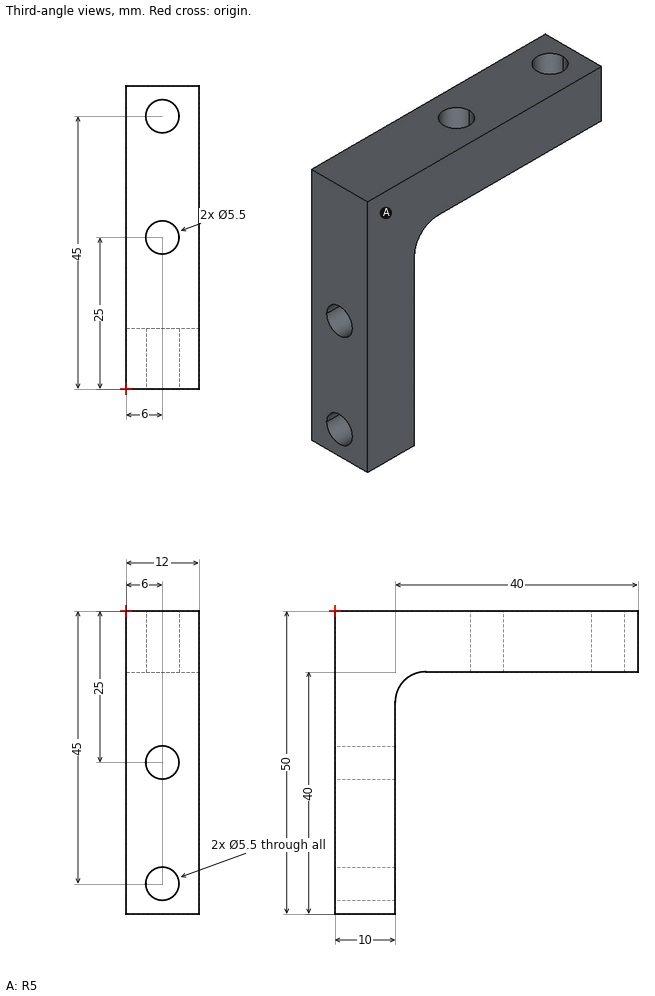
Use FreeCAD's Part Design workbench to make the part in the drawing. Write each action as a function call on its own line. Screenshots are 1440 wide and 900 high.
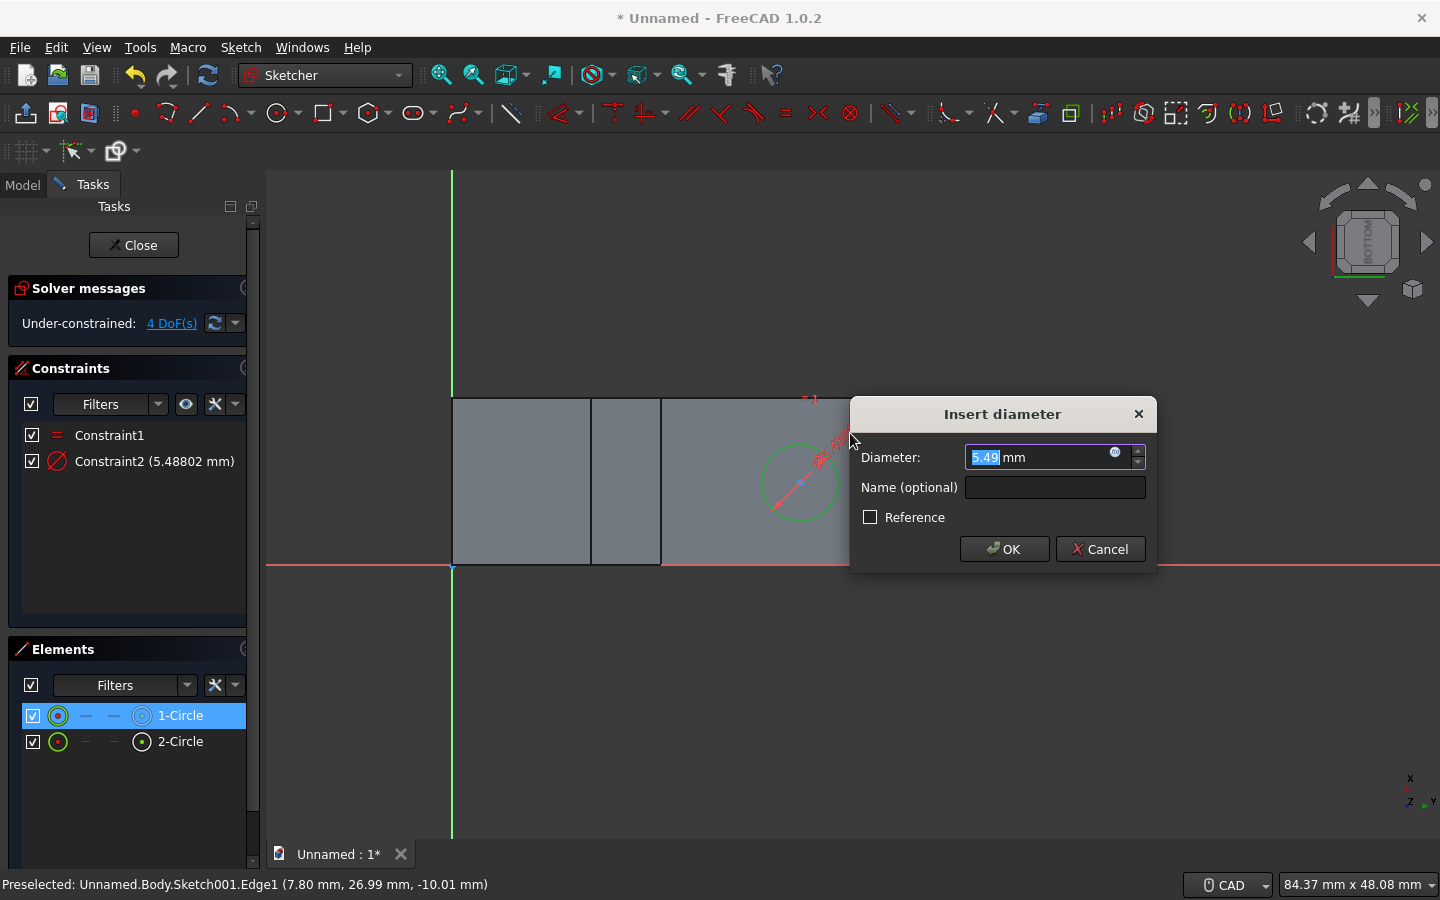
text(5.5)
key(Return)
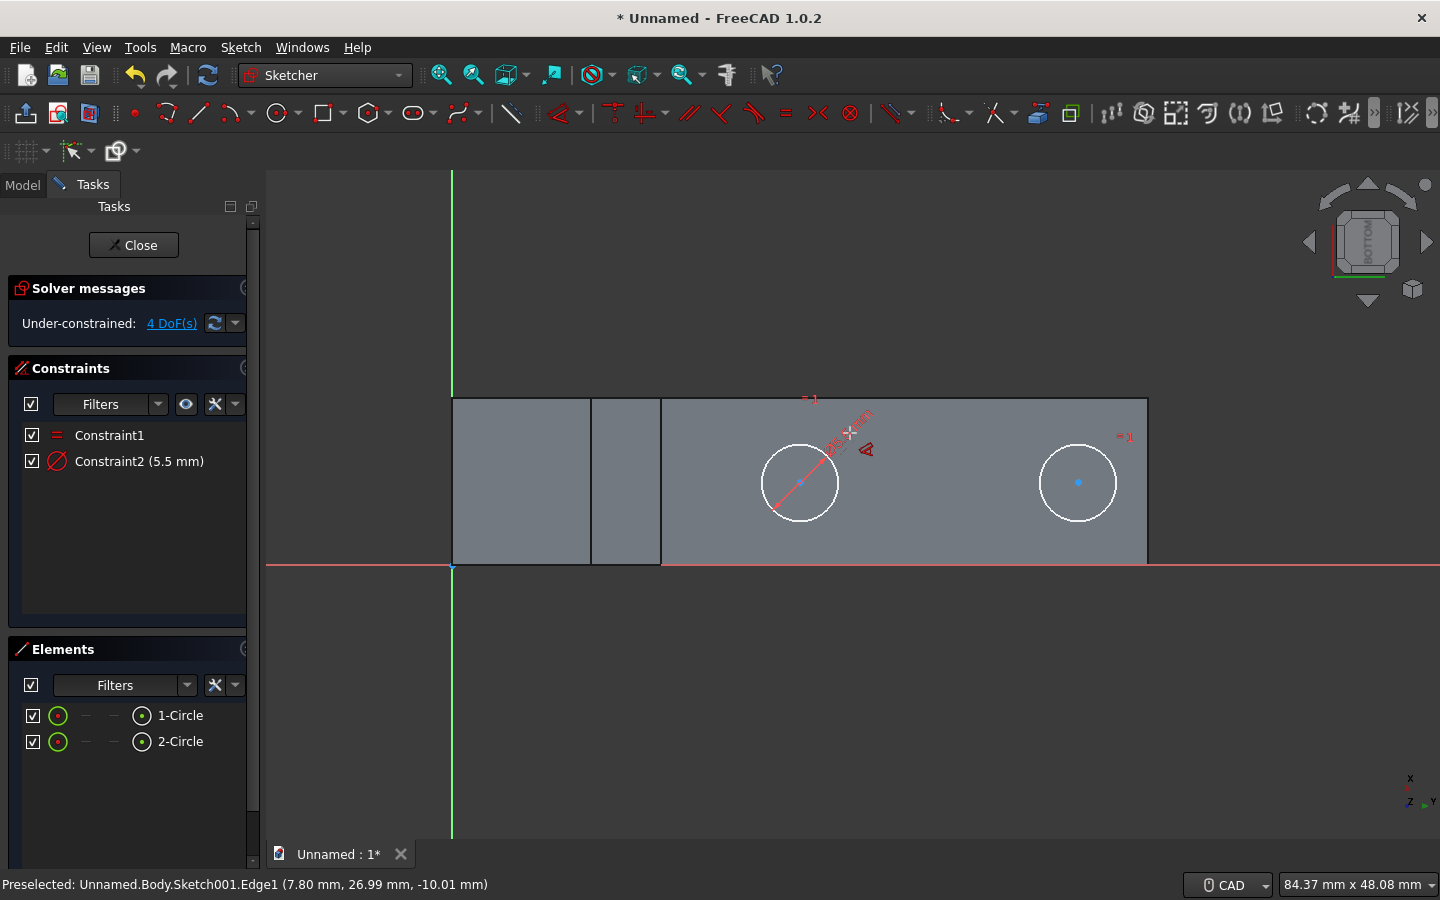
click(800, 483)
click(418, 524)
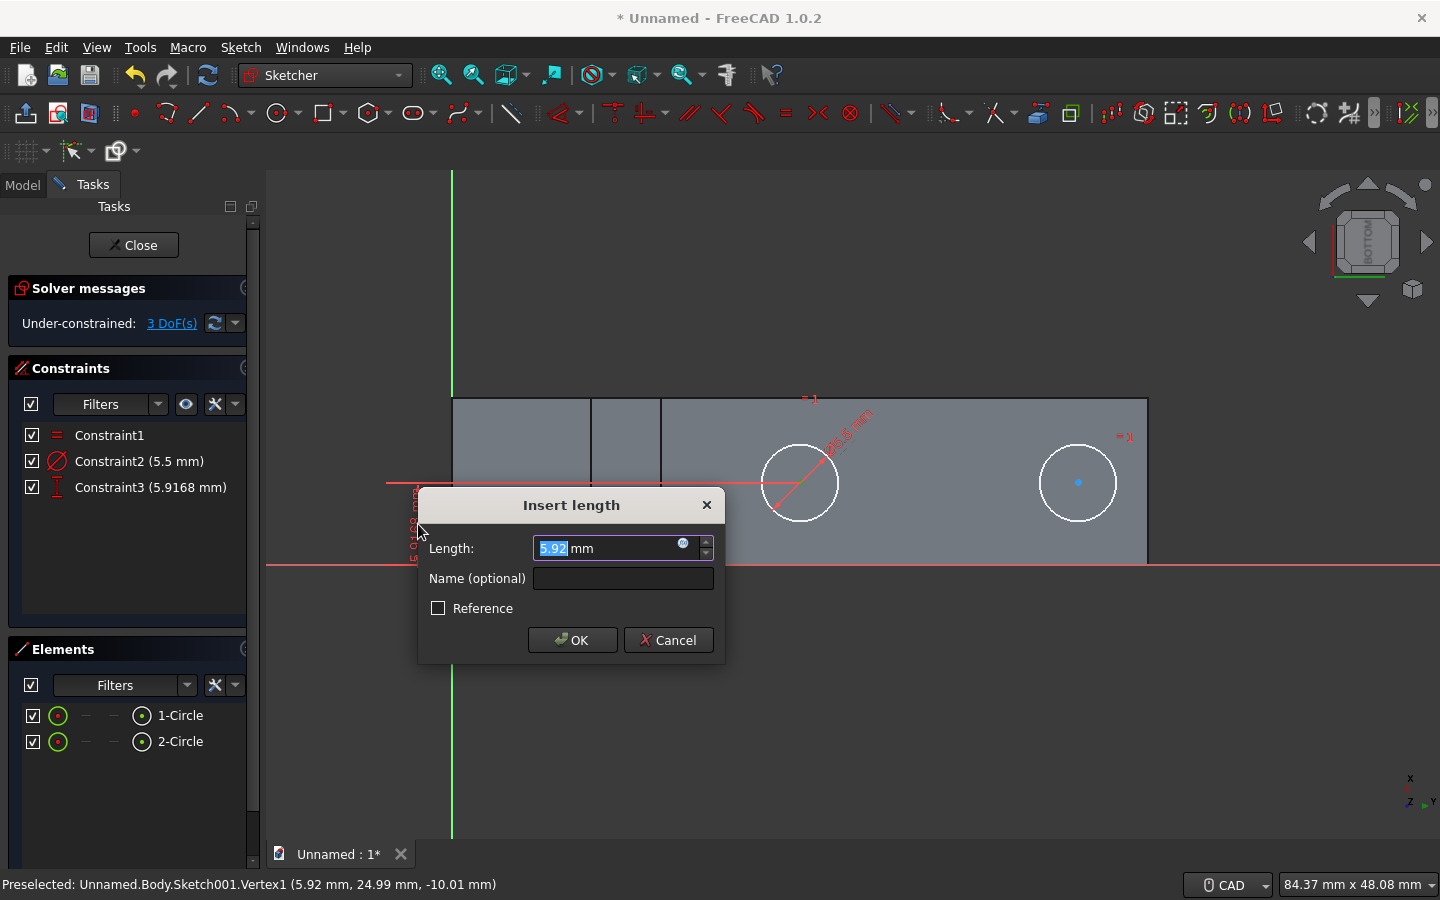
text(6)
key(Return)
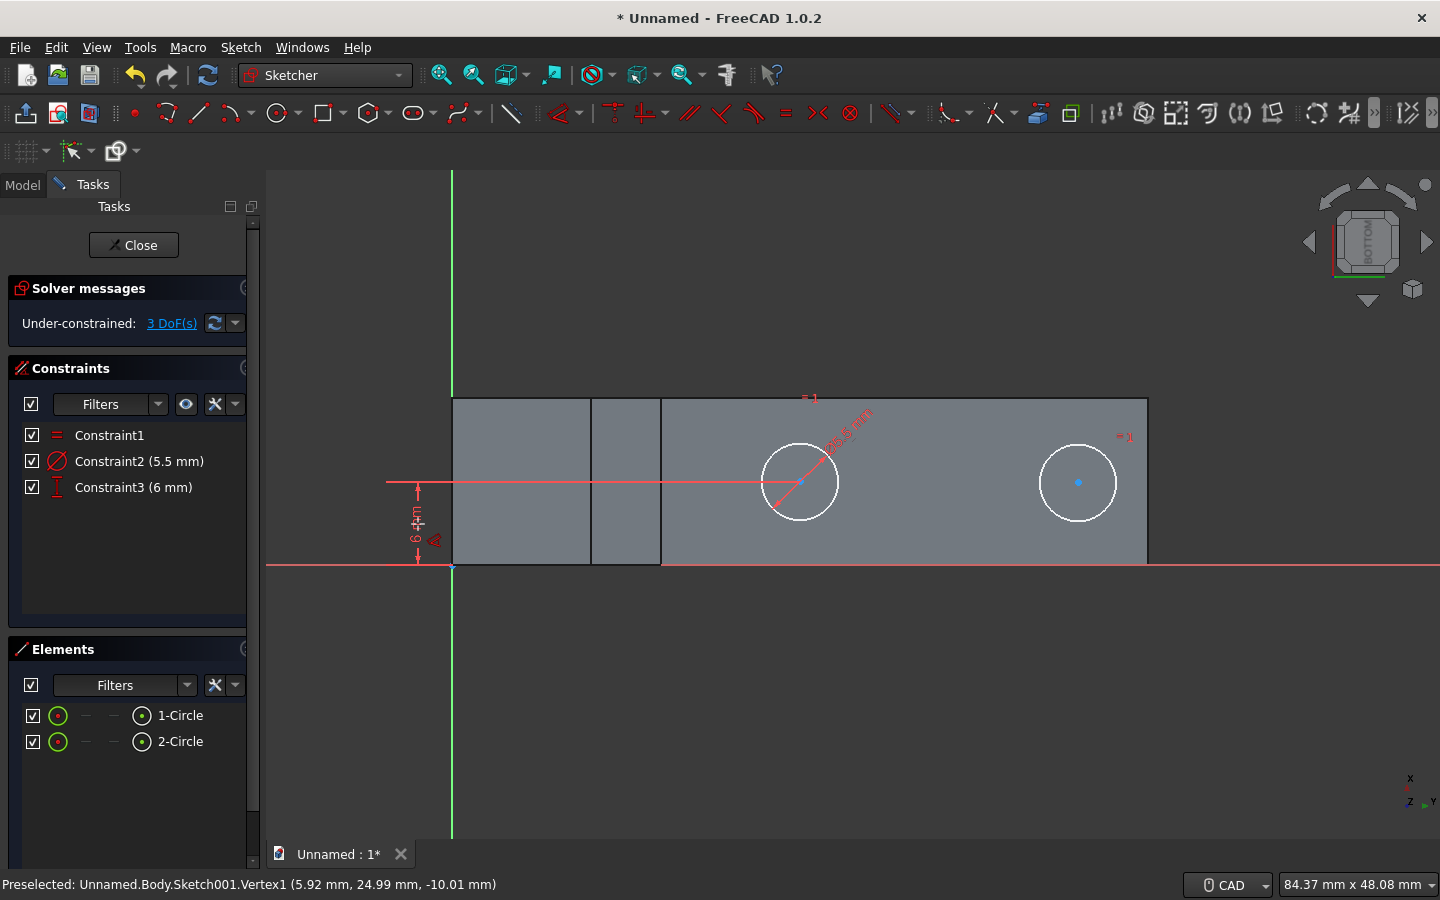
click(1078, 483)
click(418, 495)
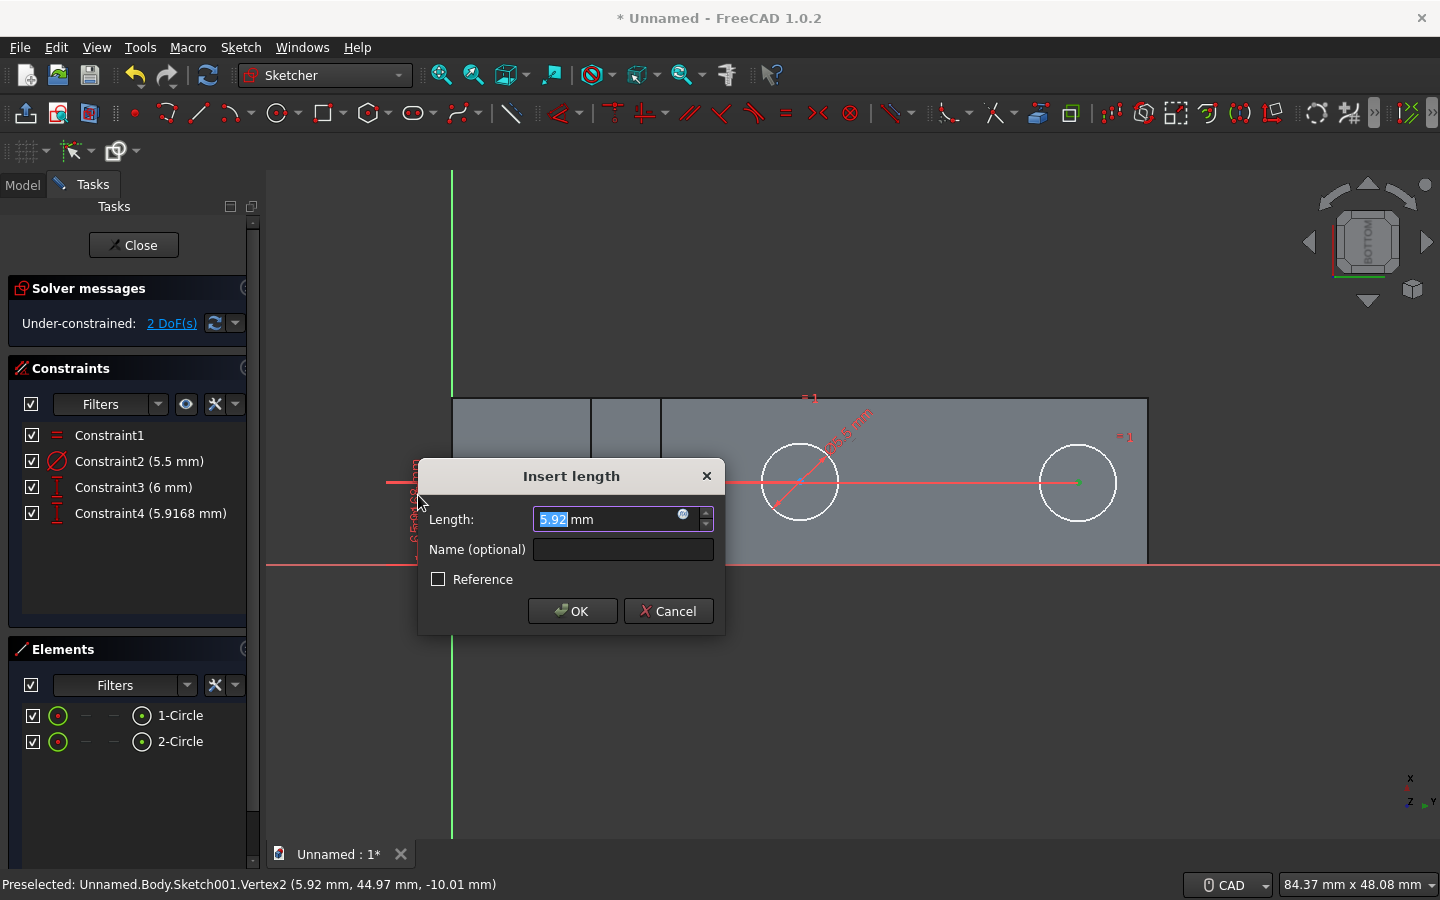
text(6)
key(Return)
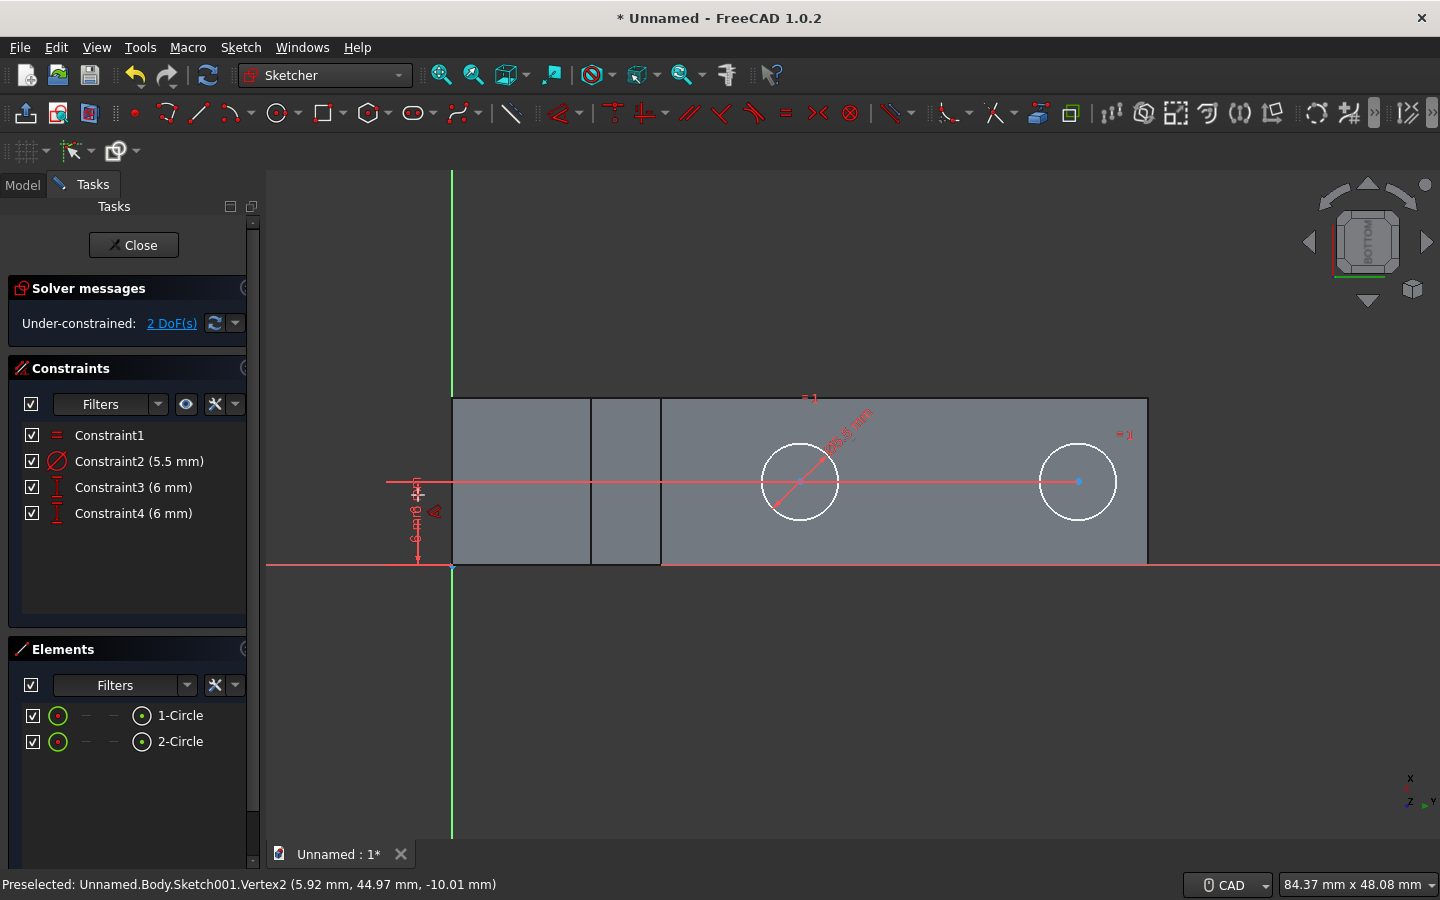
click(800, 482)
click(626, 599)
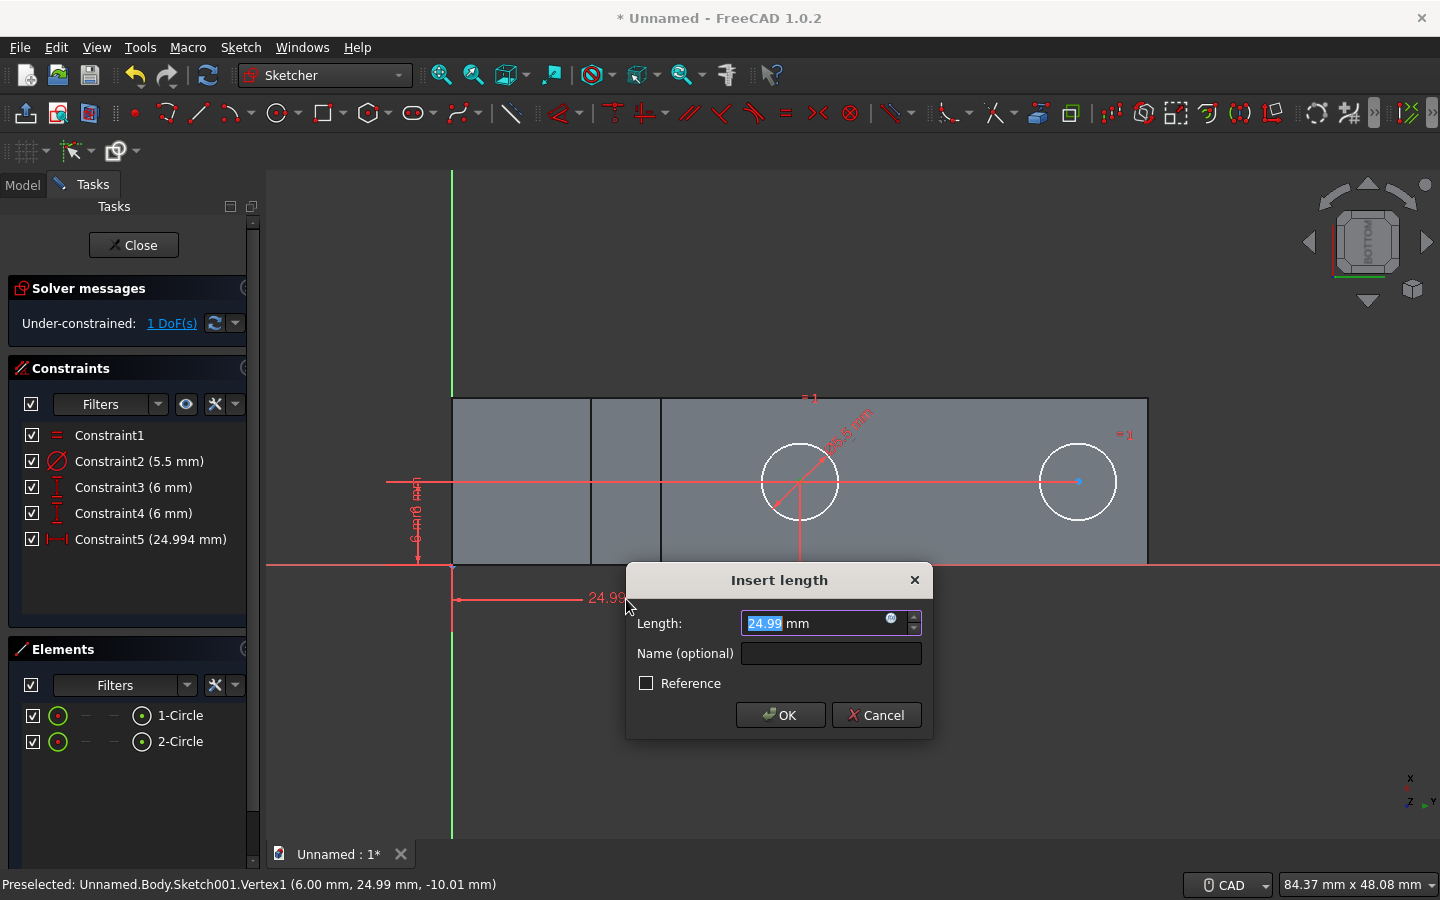
text(25)
key(Return)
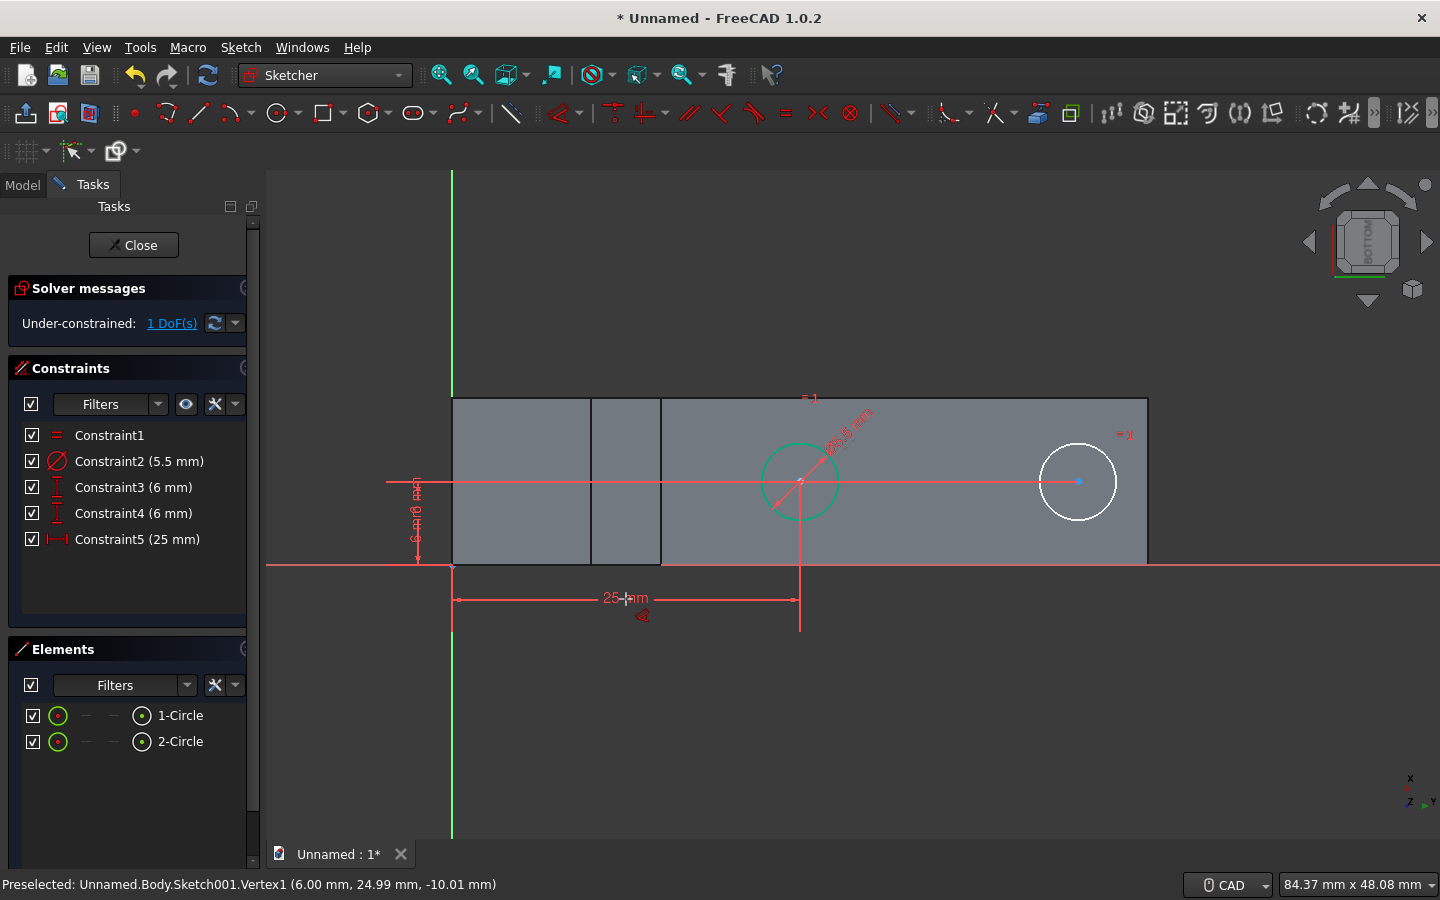
click(1078, 482)
click(765, 599)